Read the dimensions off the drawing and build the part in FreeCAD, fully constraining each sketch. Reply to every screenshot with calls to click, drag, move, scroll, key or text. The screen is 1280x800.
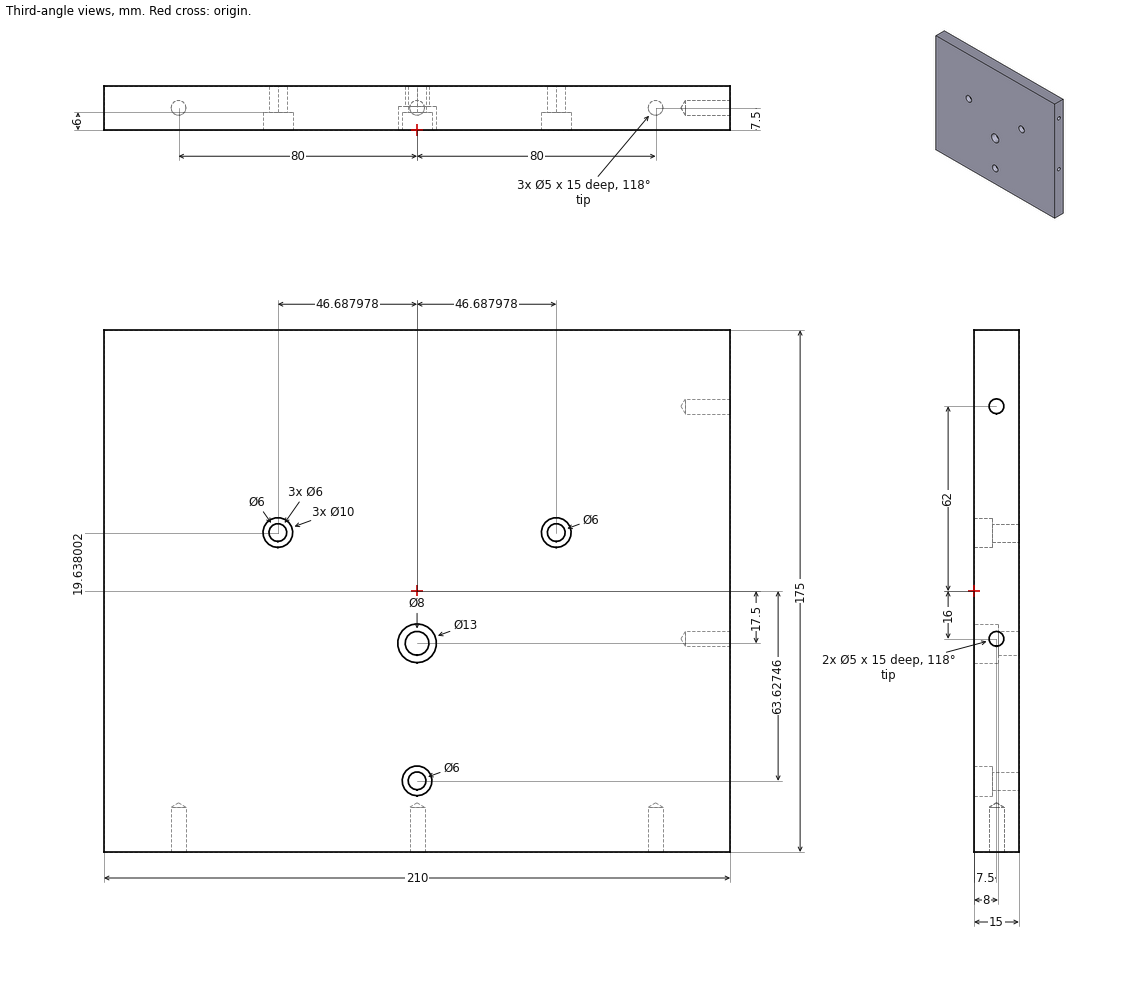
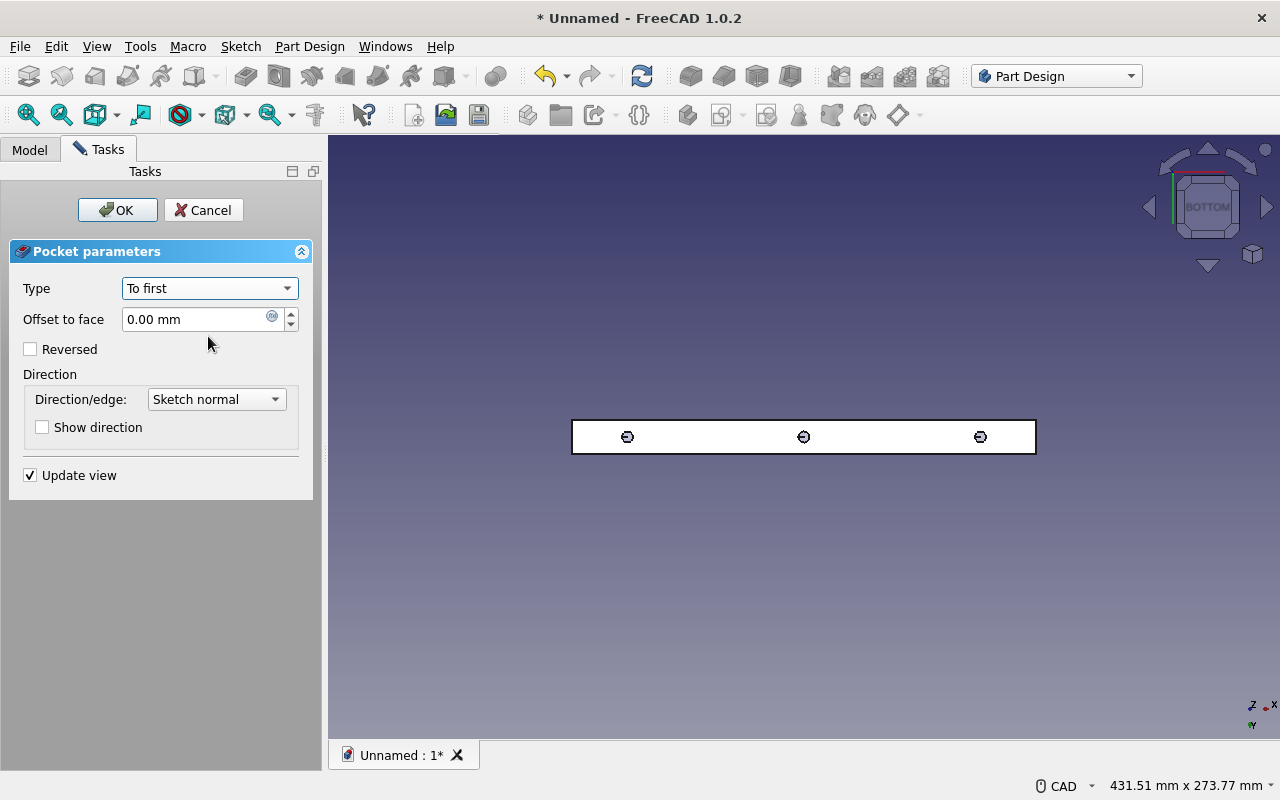
click(118, 210)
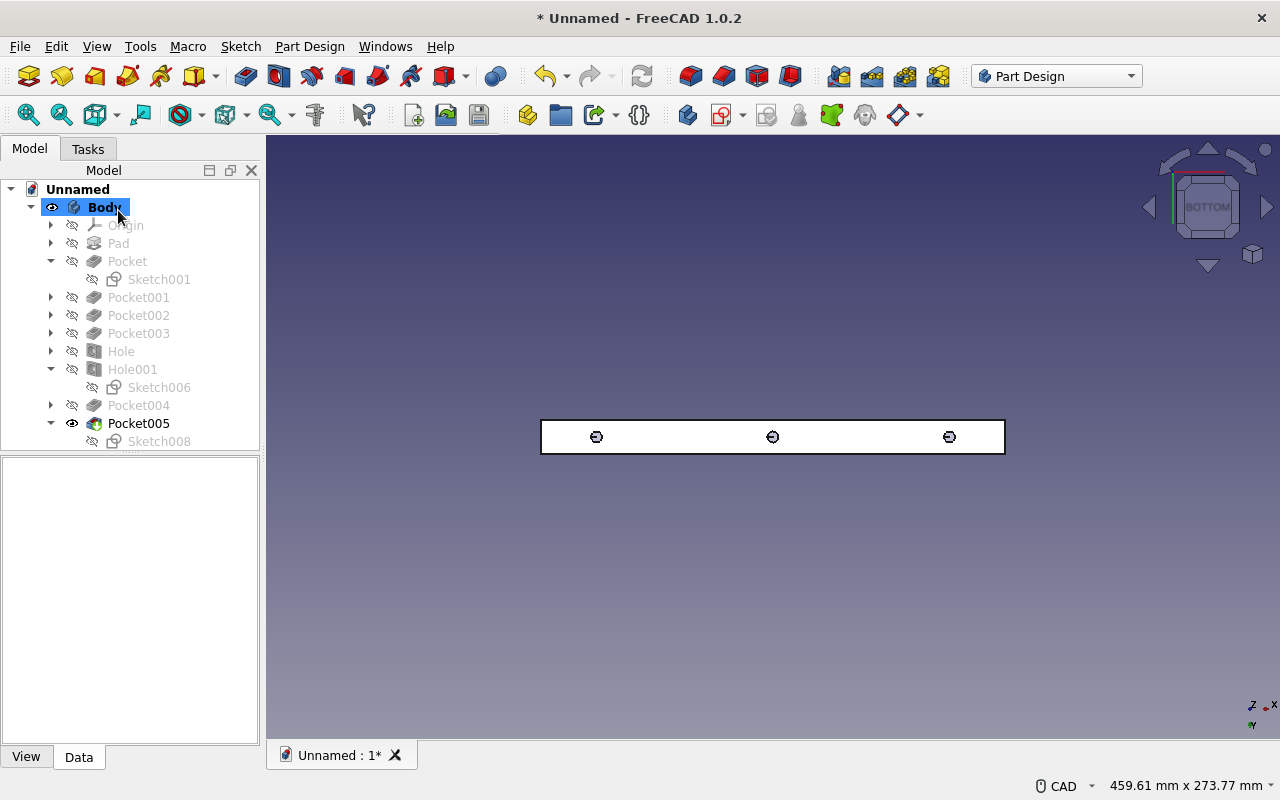
key(0)